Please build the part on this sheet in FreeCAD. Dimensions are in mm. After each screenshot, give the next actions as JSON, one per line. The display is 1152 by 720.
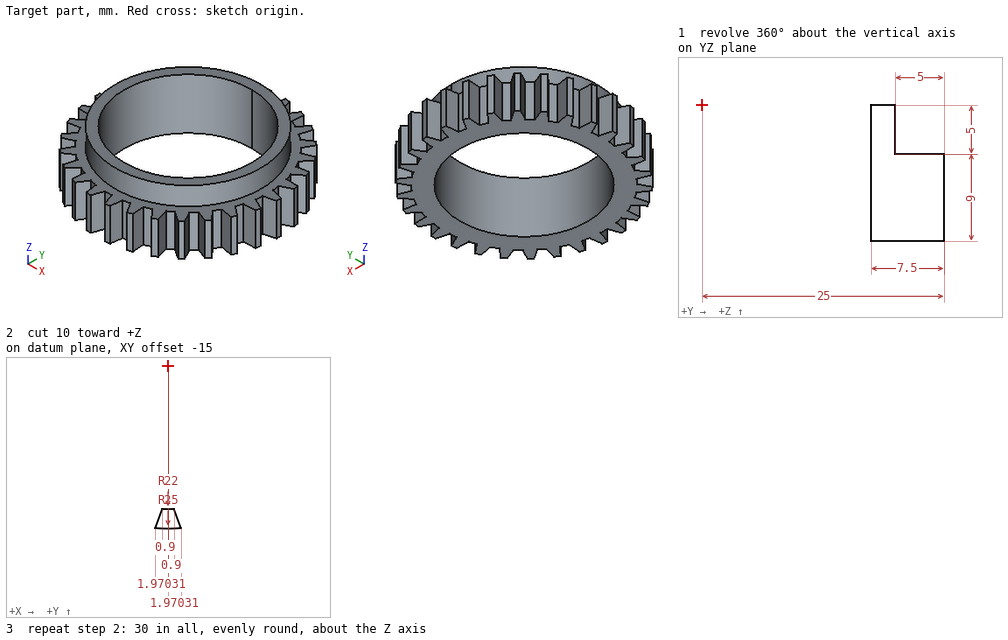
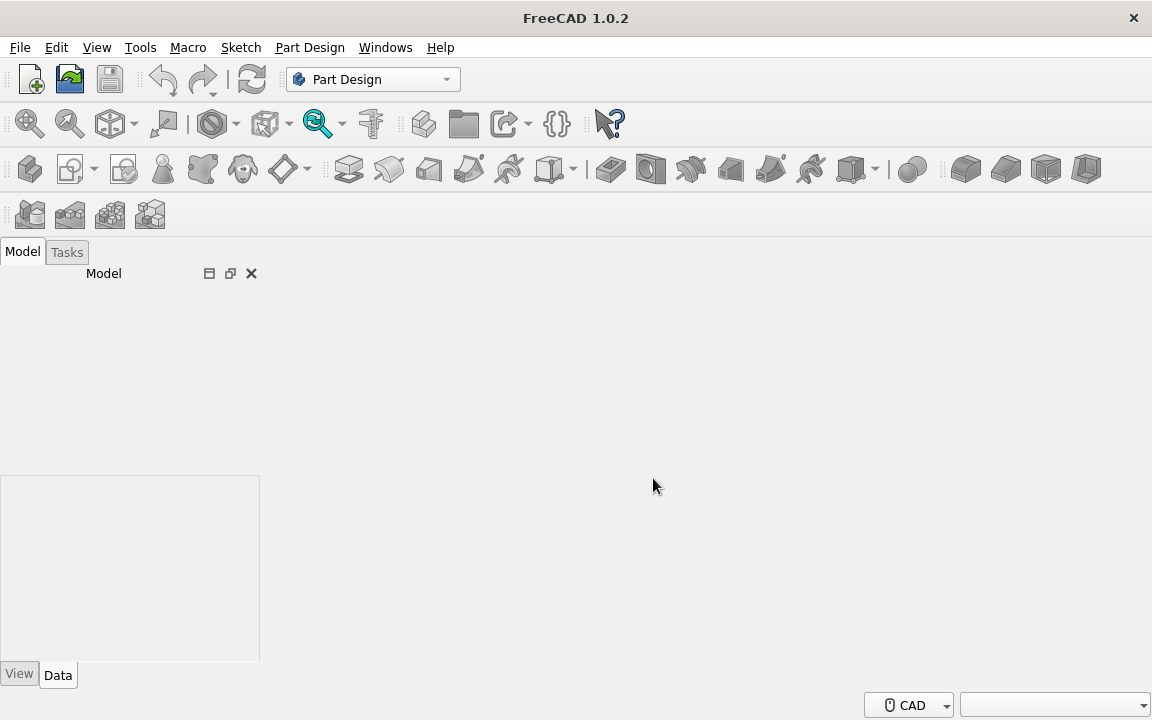
{"action": "left_click", "coordinate": [30, 80]}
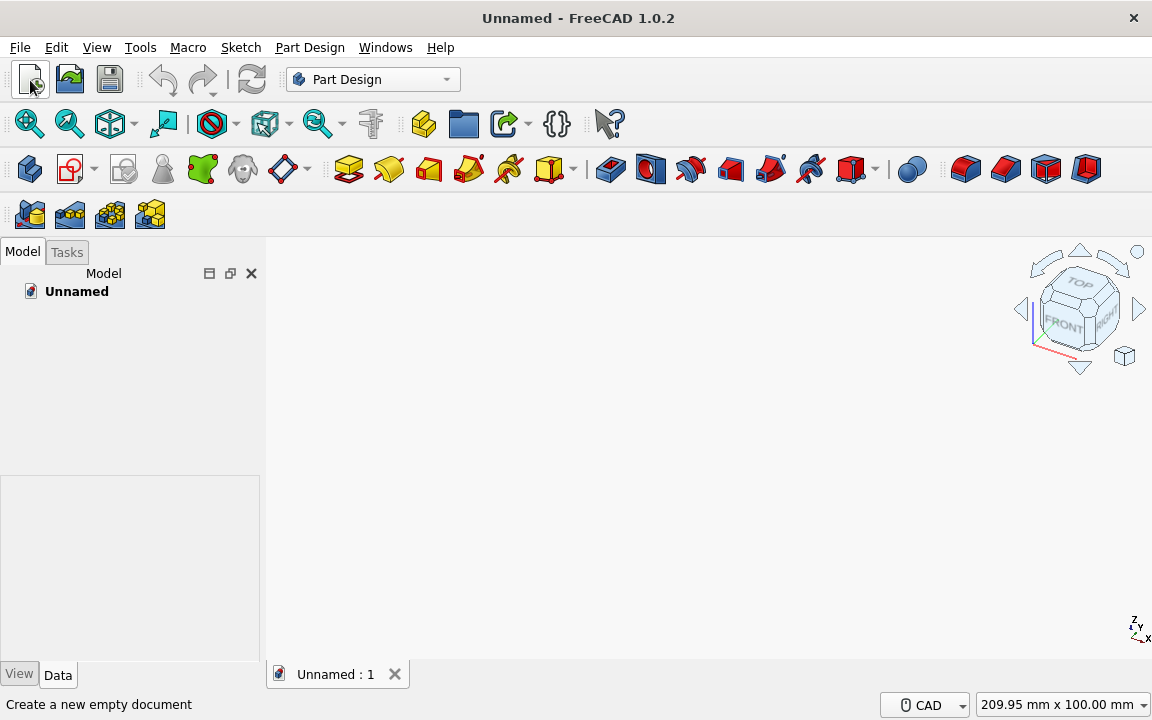
{"action": "left_click", "coordinate": [70, 170]}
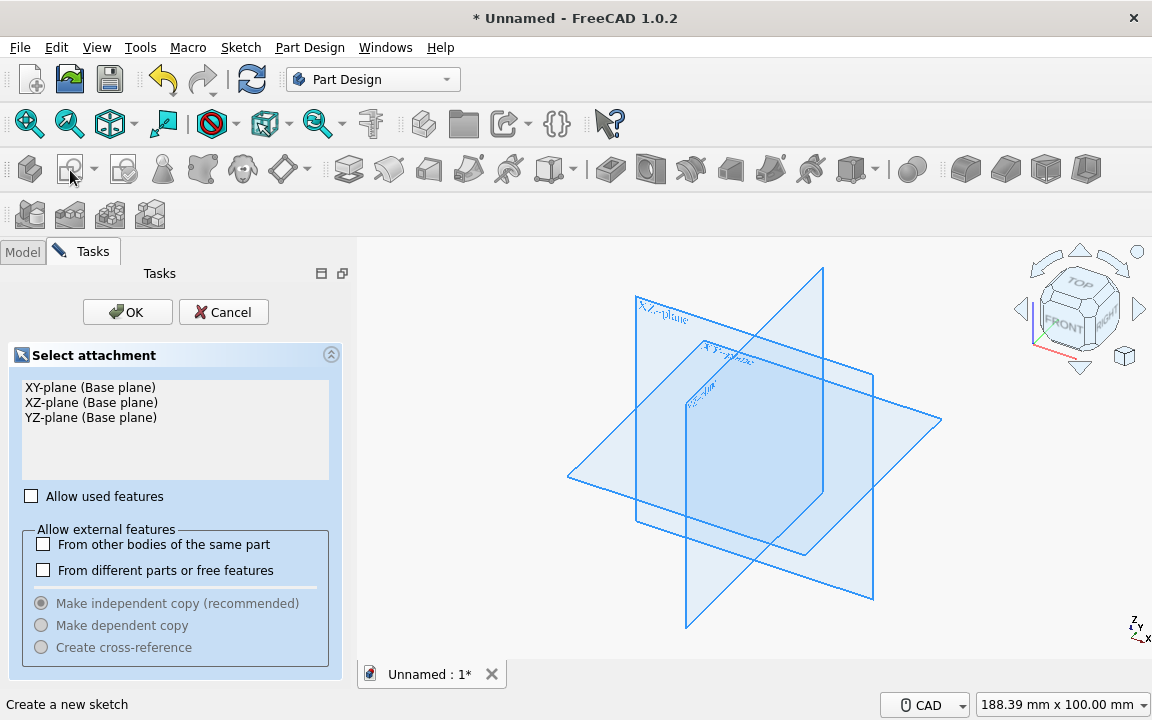
{"action": "left_click", "coordinate": [82, 418]}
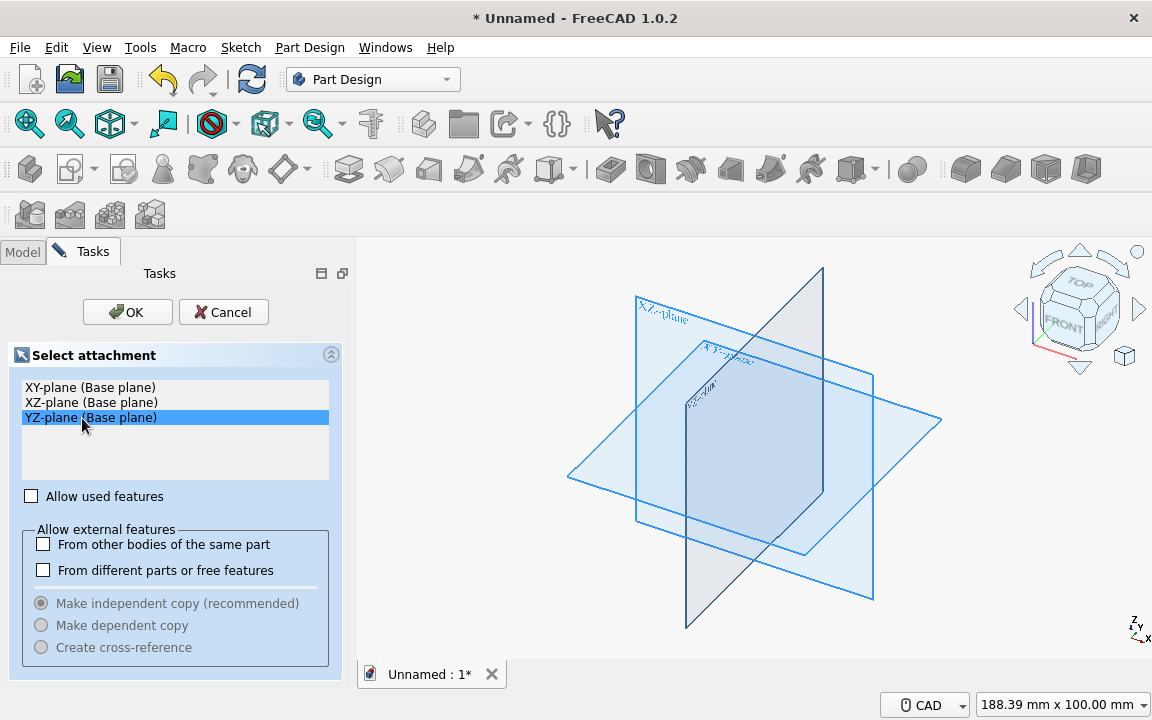
{"action": "left_click", "coordinate": [128, 312]}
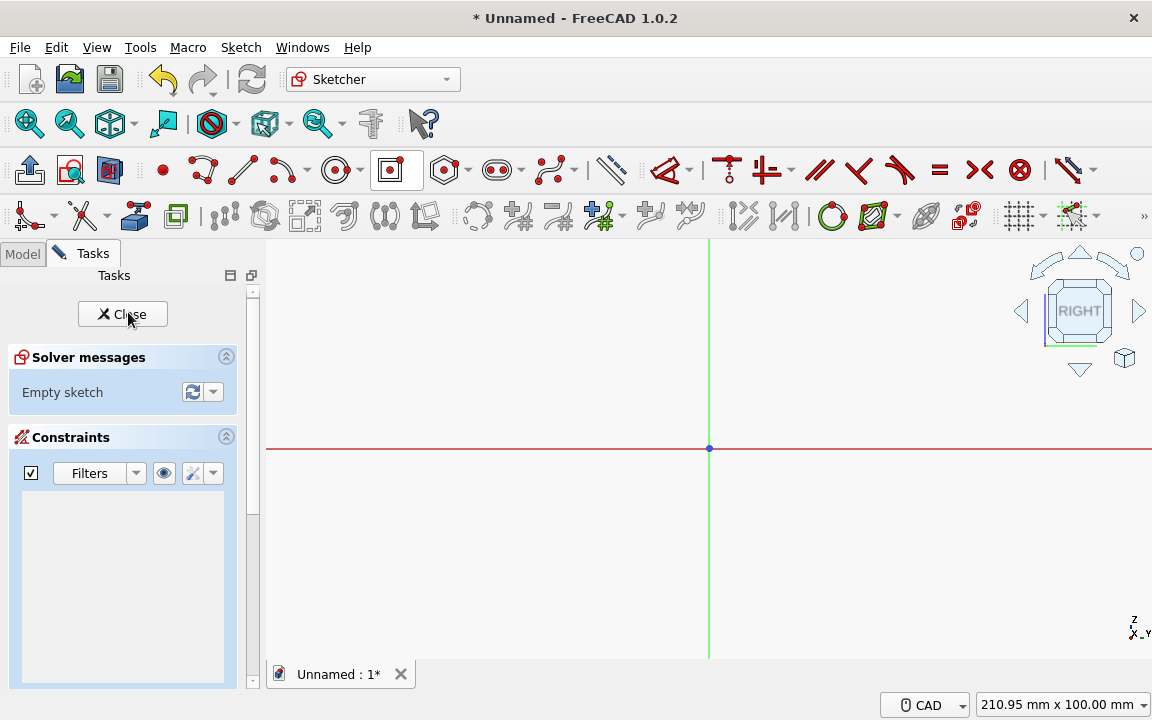
{"action": "scroll", "coordinate": [801, 488], "scroll_direction": "up", "scroll_amount": 7}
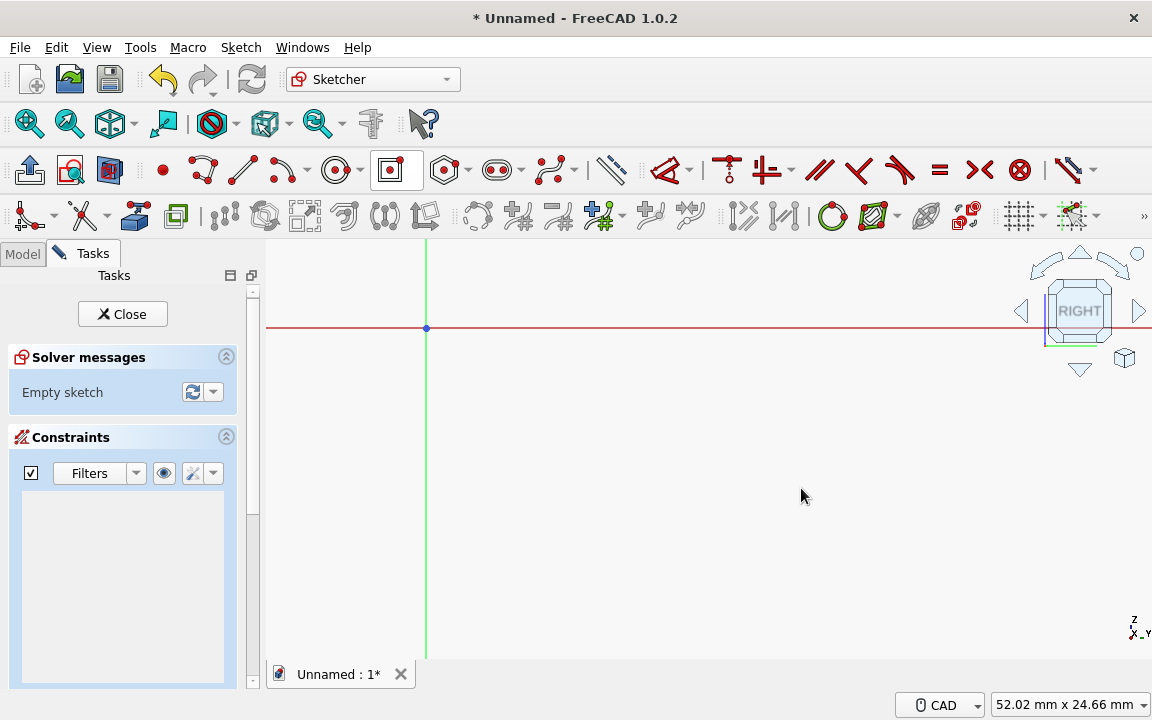
{"action": "left_click", "coordinate": [204, 170]}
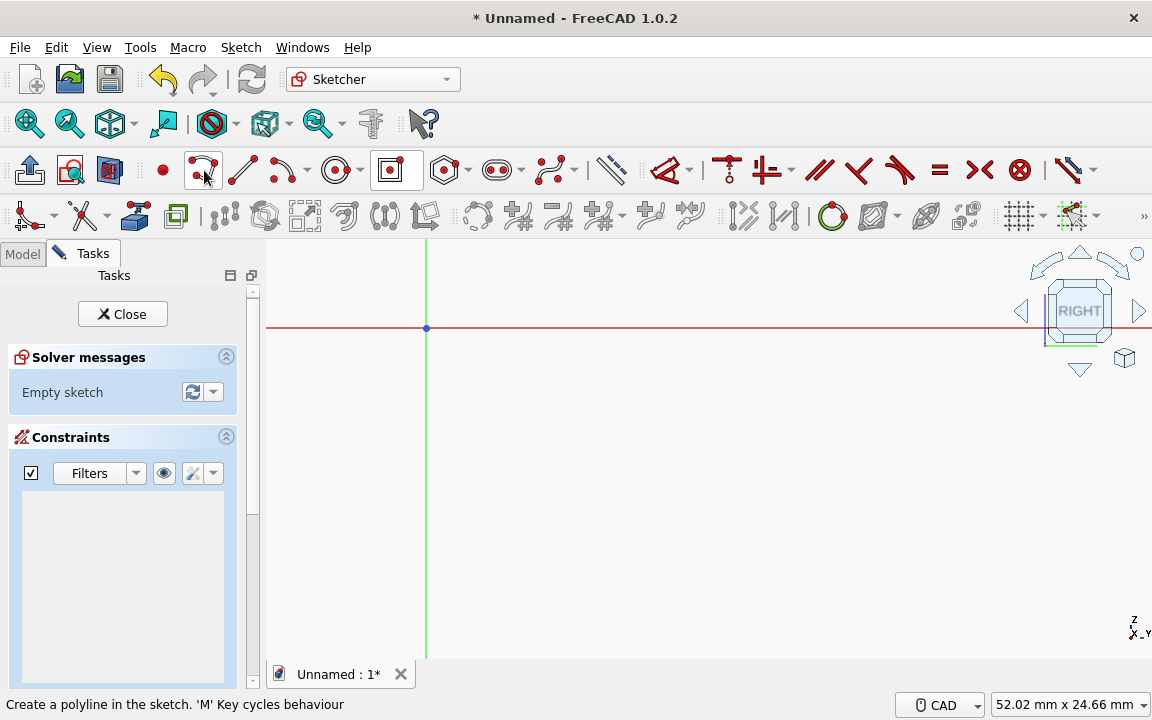
{"action": "left_click", "coordinate": [724, 328]}
{"action": "left_click", "coordinate": [724, 566]}
{"action": "left_click", "coordinate": [852, 566]}
{"action": "left_click", "coordinate": [852, 413]}
{"action": "left_click", "coordinate": [767, 413]}
{"action": "left_click", "coordinate": [767, 337]}
{"action": "left_click", "coordinate": [724, 328]}
{"action": "key", "text": "Escape"}
{"action": "key", "text": "Escape"}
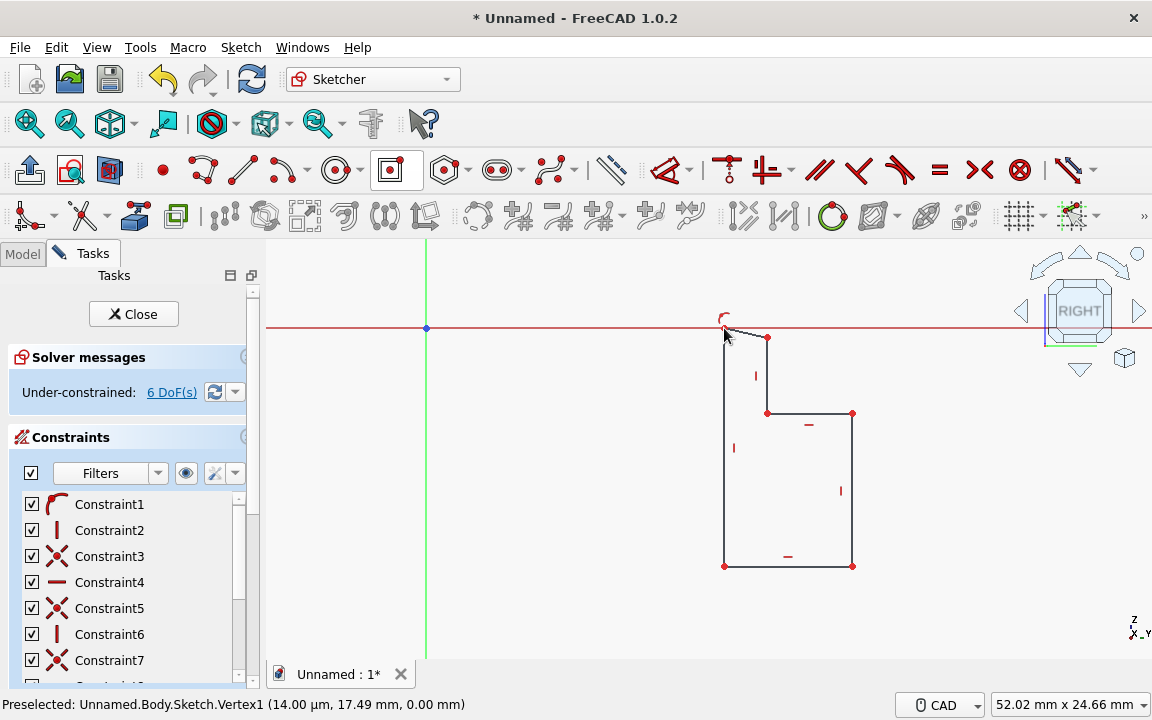
{"action": "left_click", "coordinate": [737, 331]}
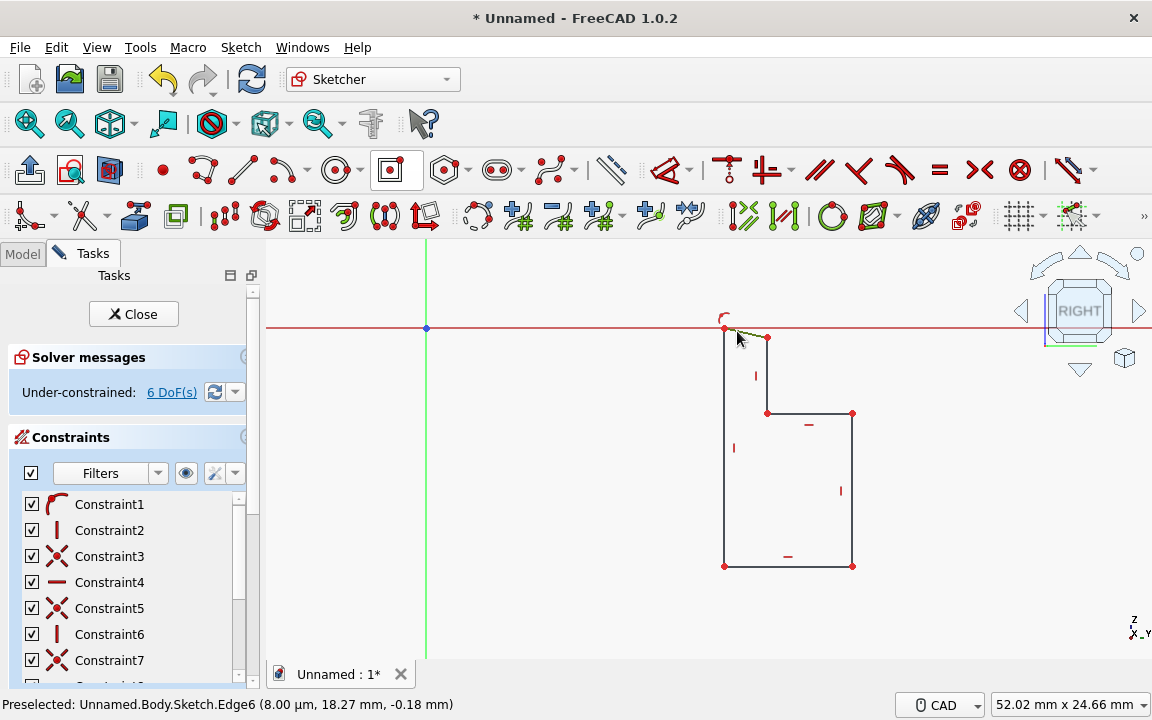
{"action": "key", "text": "h"}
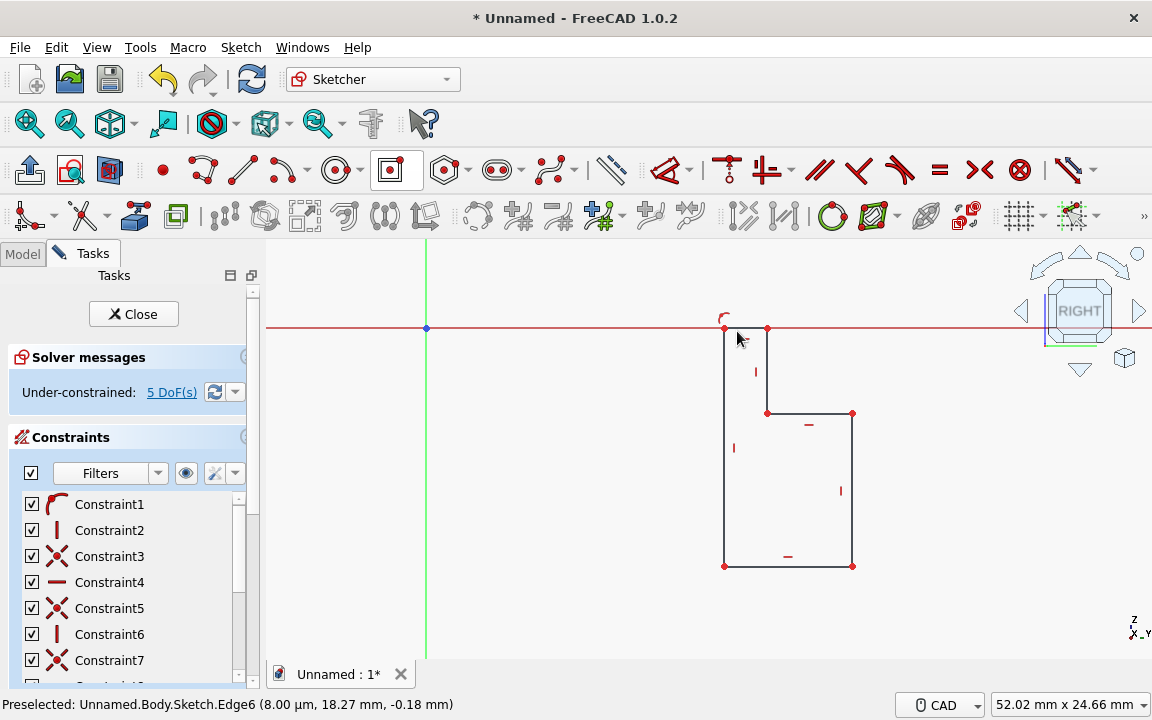
{"action": "left_click", "coordinate": [666, 170]}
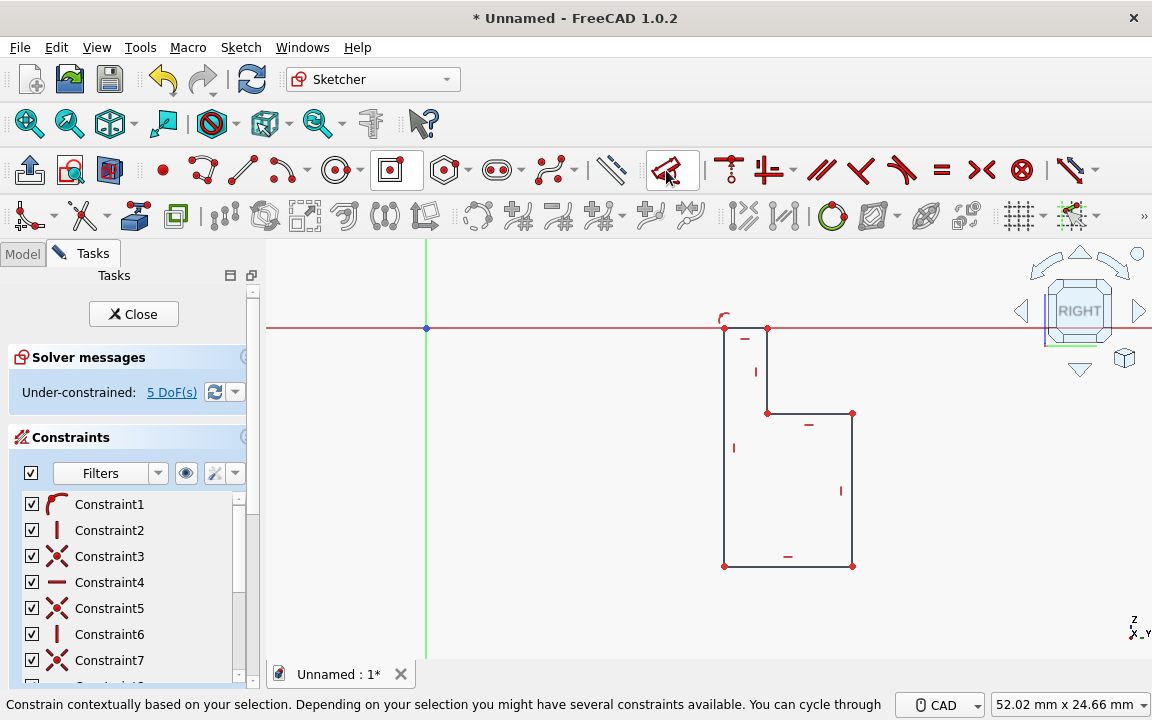
{"action": "left_click", "coordinate": [852, 521]}
{"action": "left_click", "coordinate": [886, 491]}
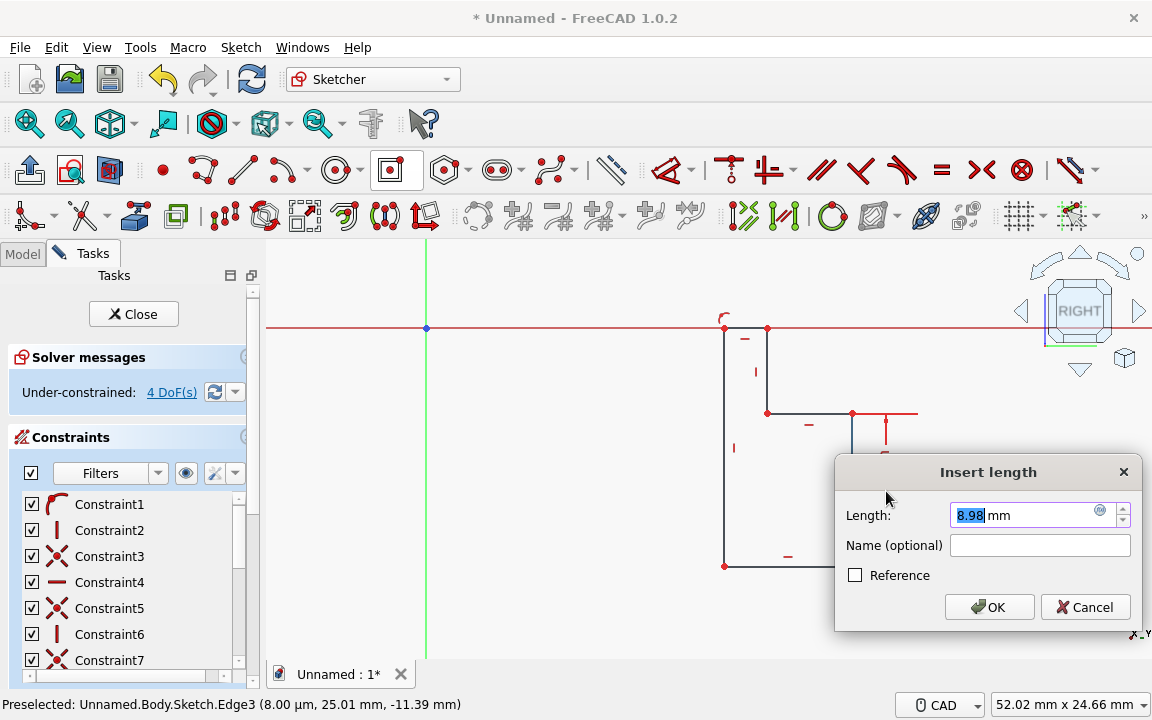
{"action": "type", "text": "9"}
{"action": "key", "text": "Return"}